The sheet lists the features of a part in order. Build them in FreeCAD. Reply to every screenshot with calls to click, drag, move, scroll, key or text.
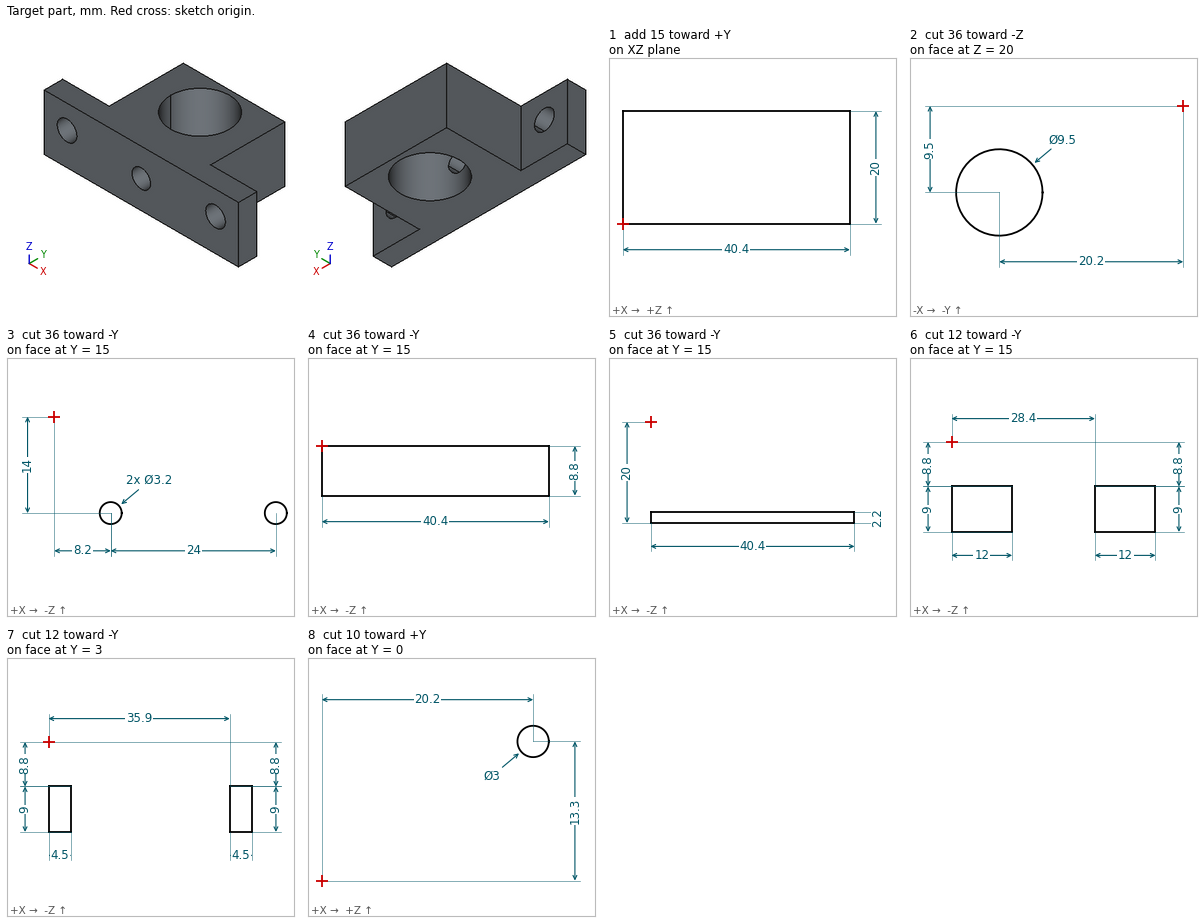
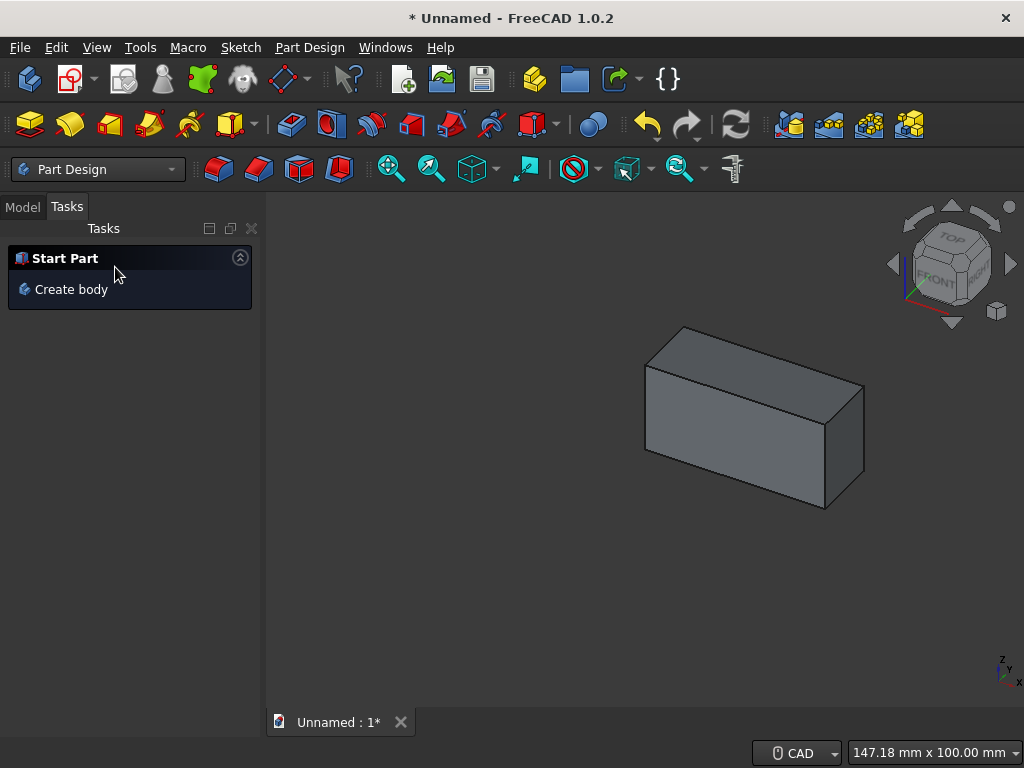
key(v)
key(f)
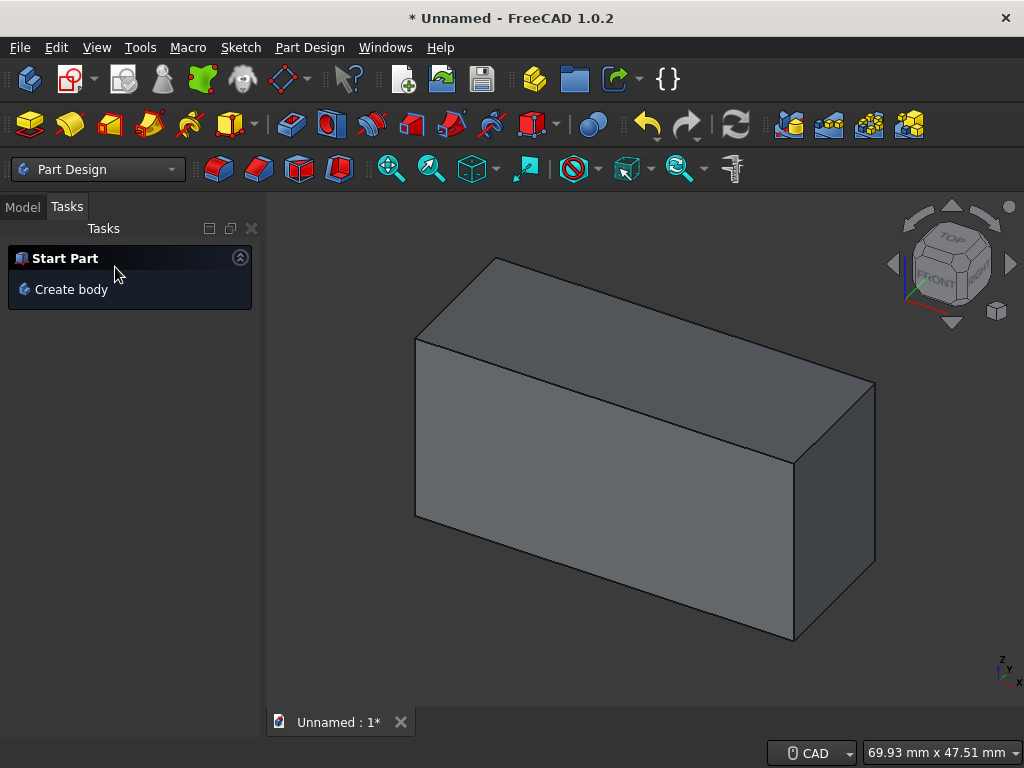
click(753, 396)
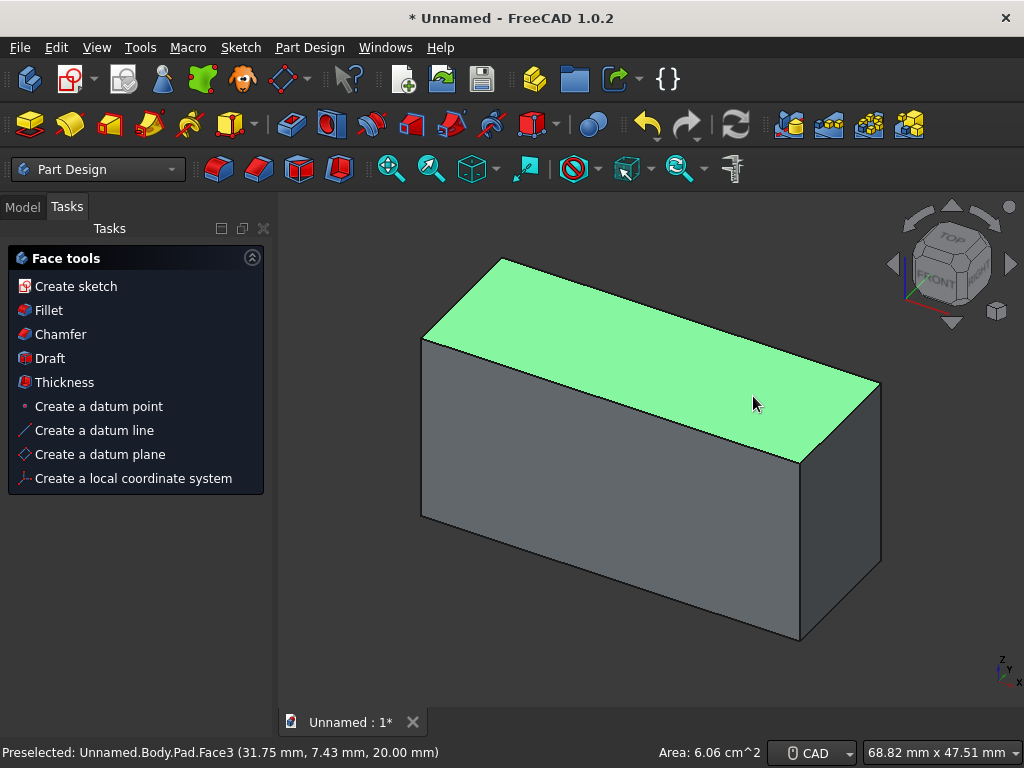
click(70, 80)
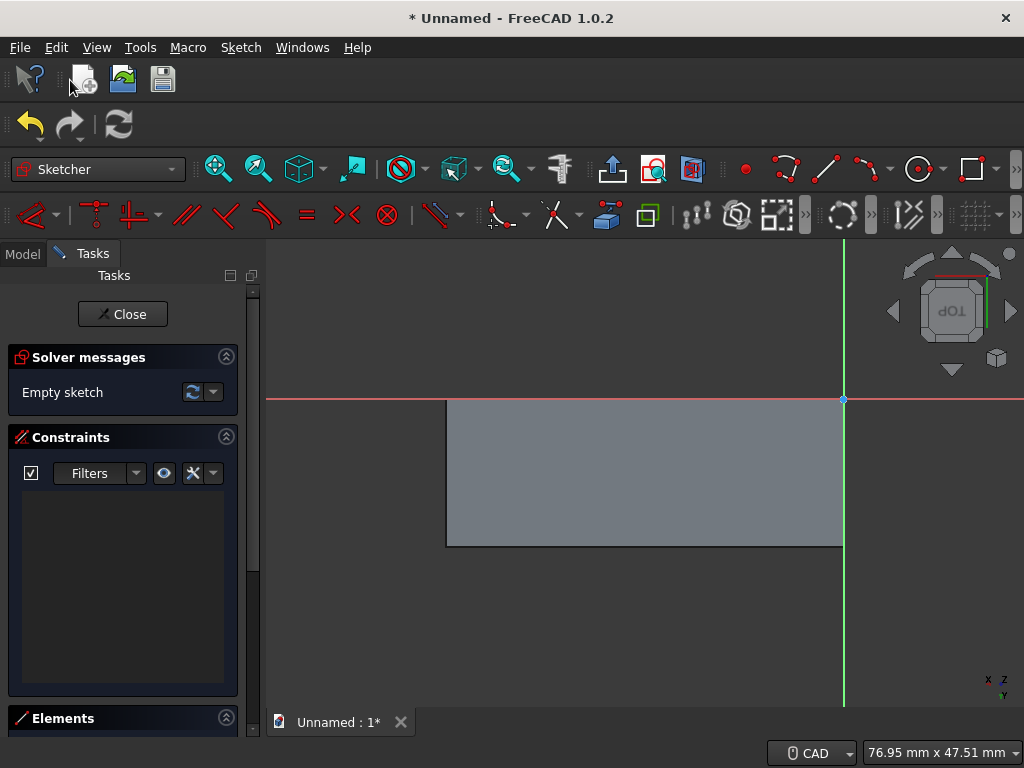
scroll(675, 501, up, 6)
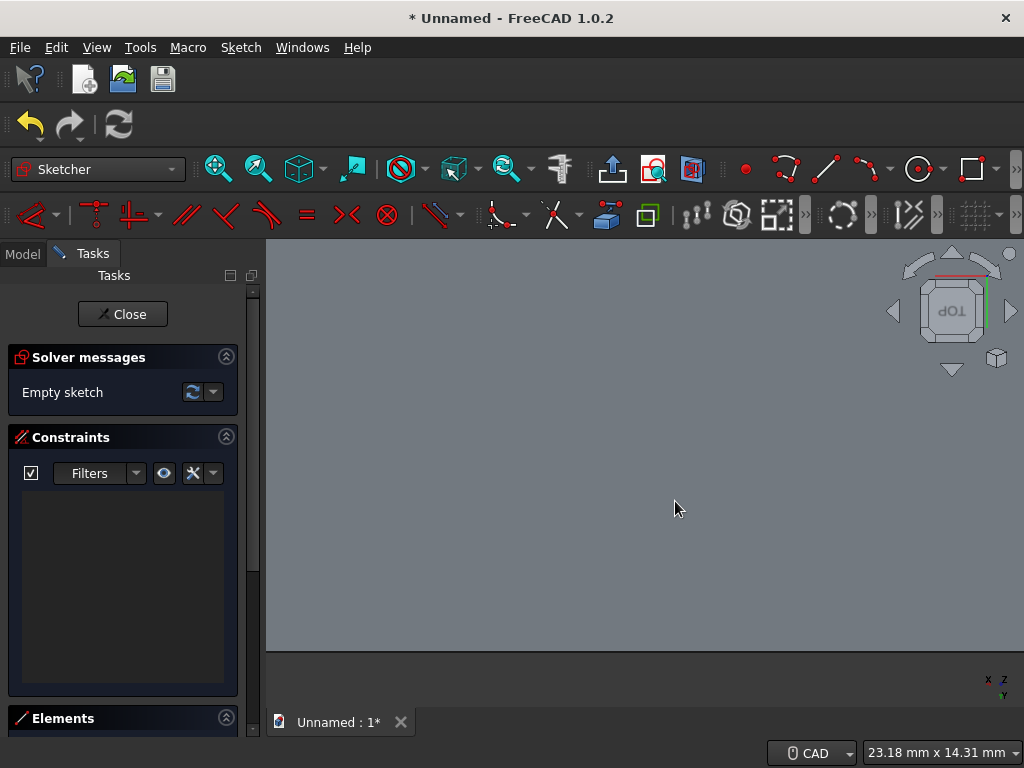
click(920, 170)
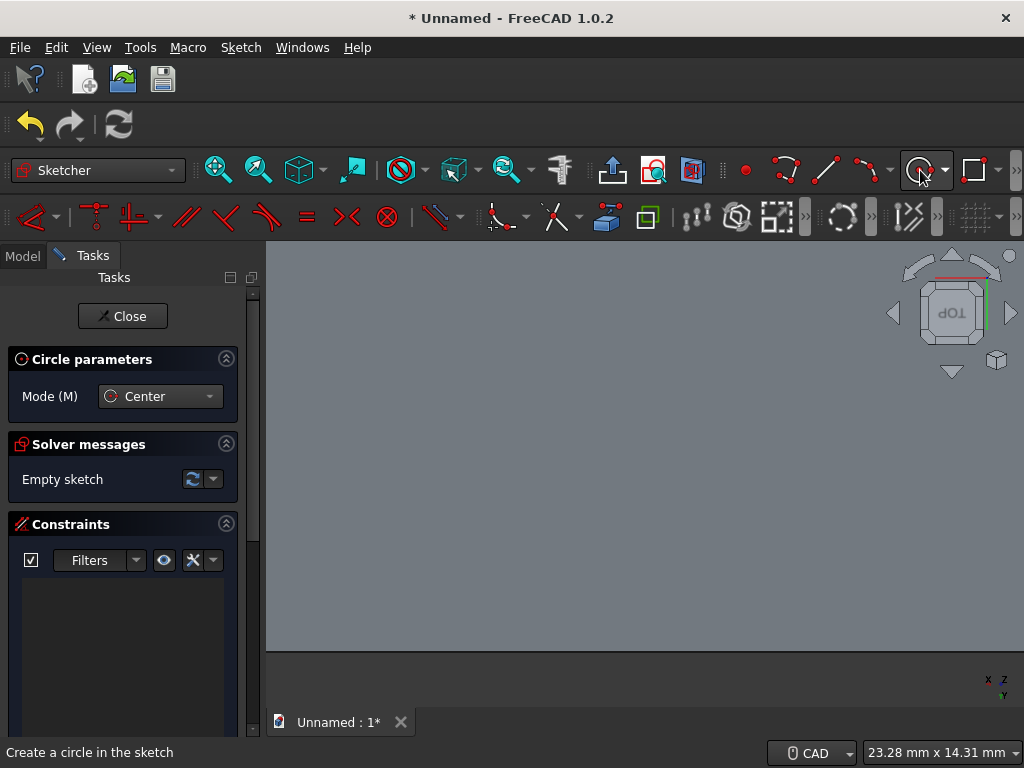
click(574, 473)
move(684, 364)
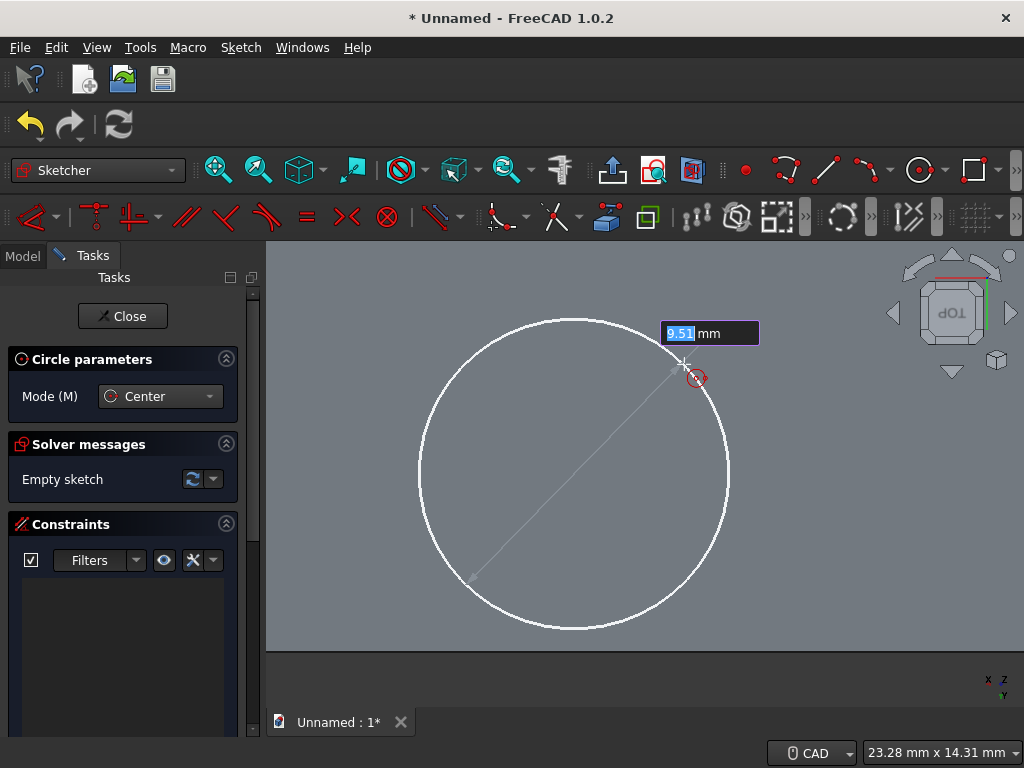
text(9.5)
key(Return)
key(Escape)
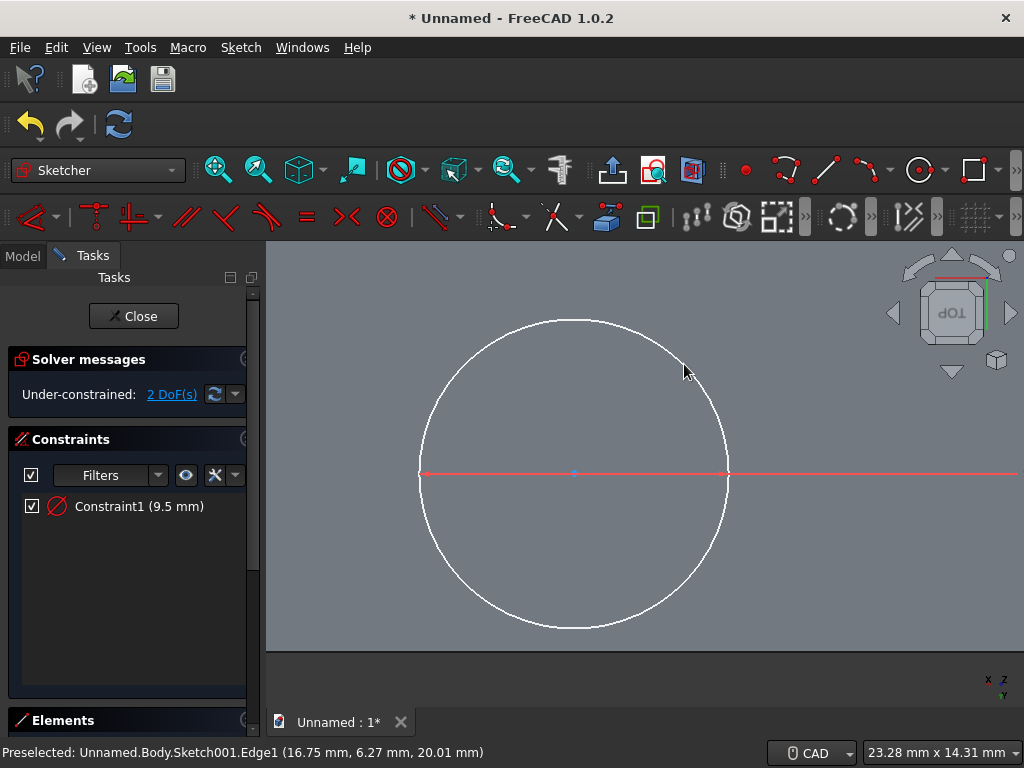
click(574, 474)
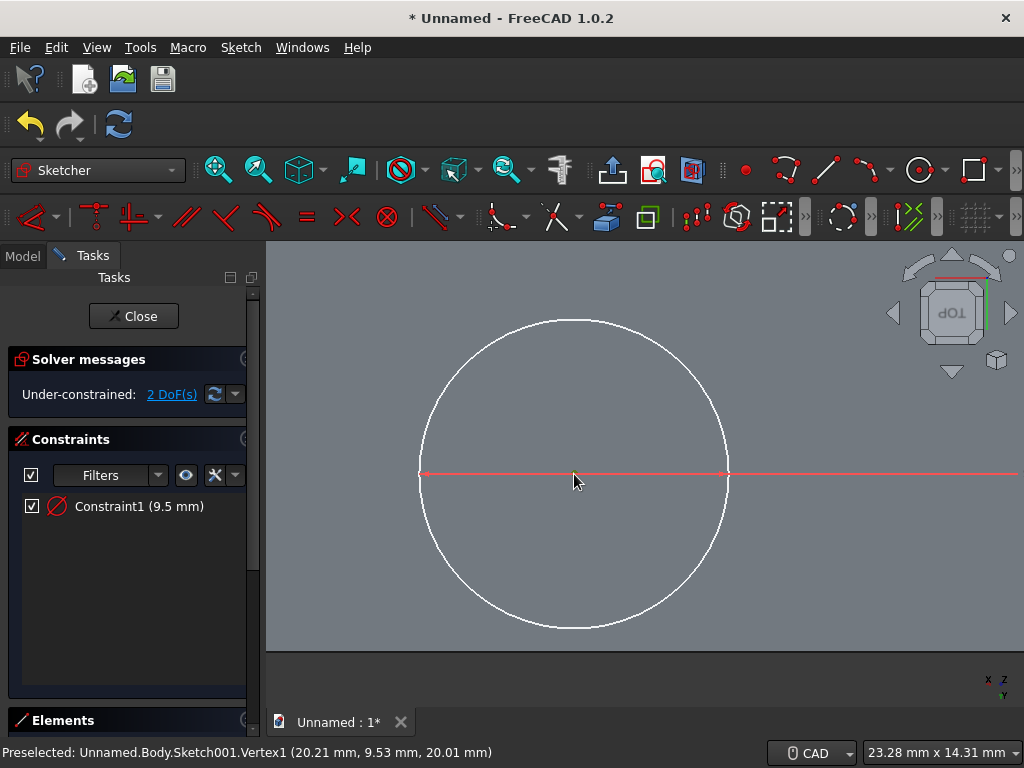
key(i)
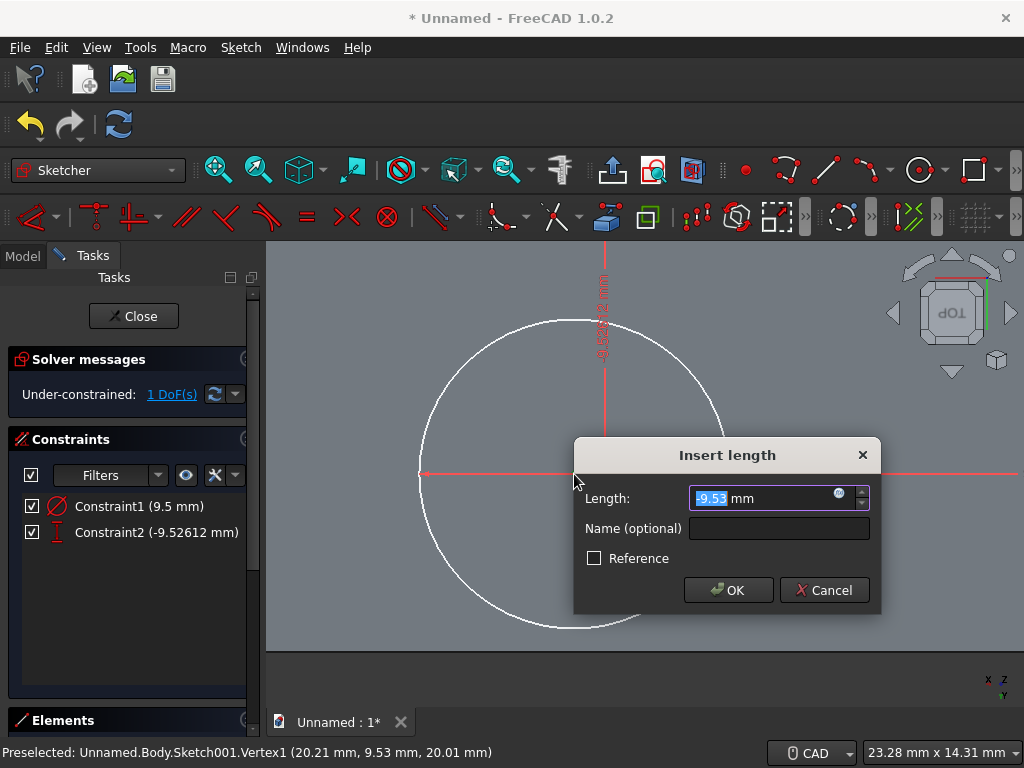
text(-9.5)
key(Return)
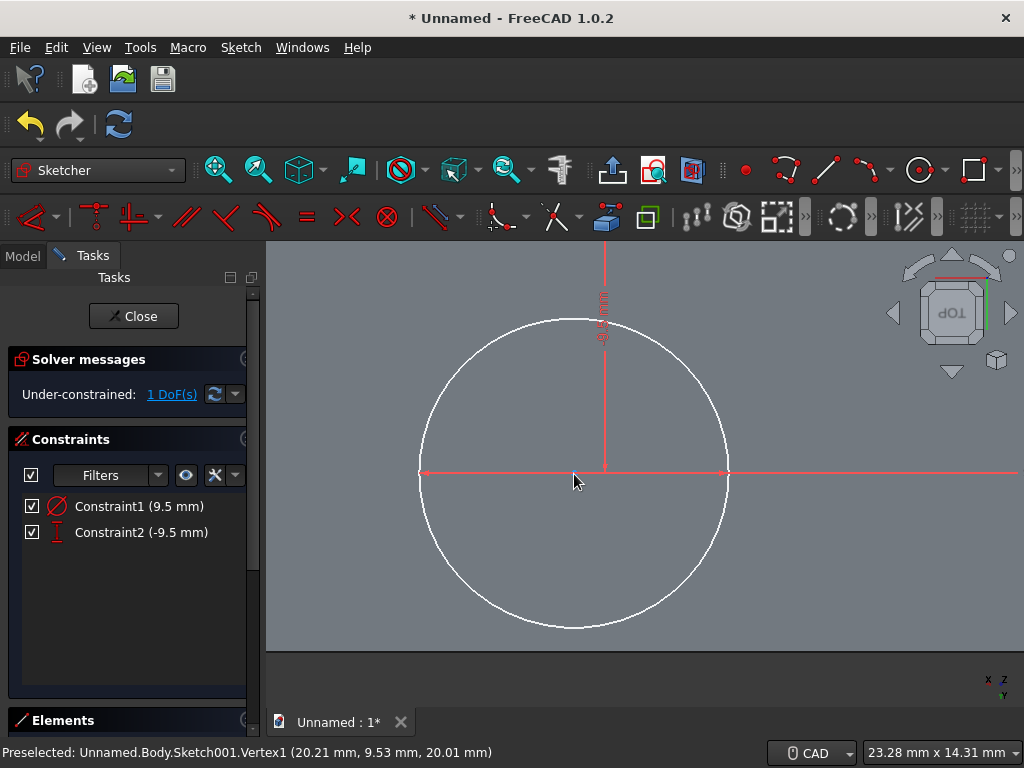
click(574, 473)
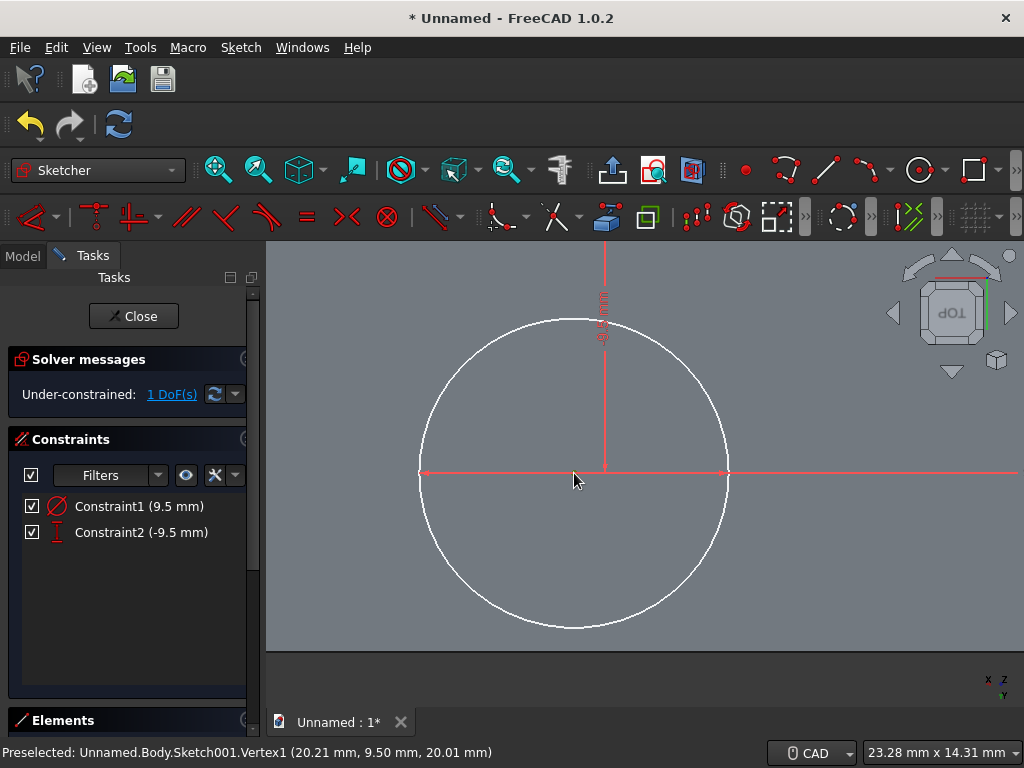
key(l)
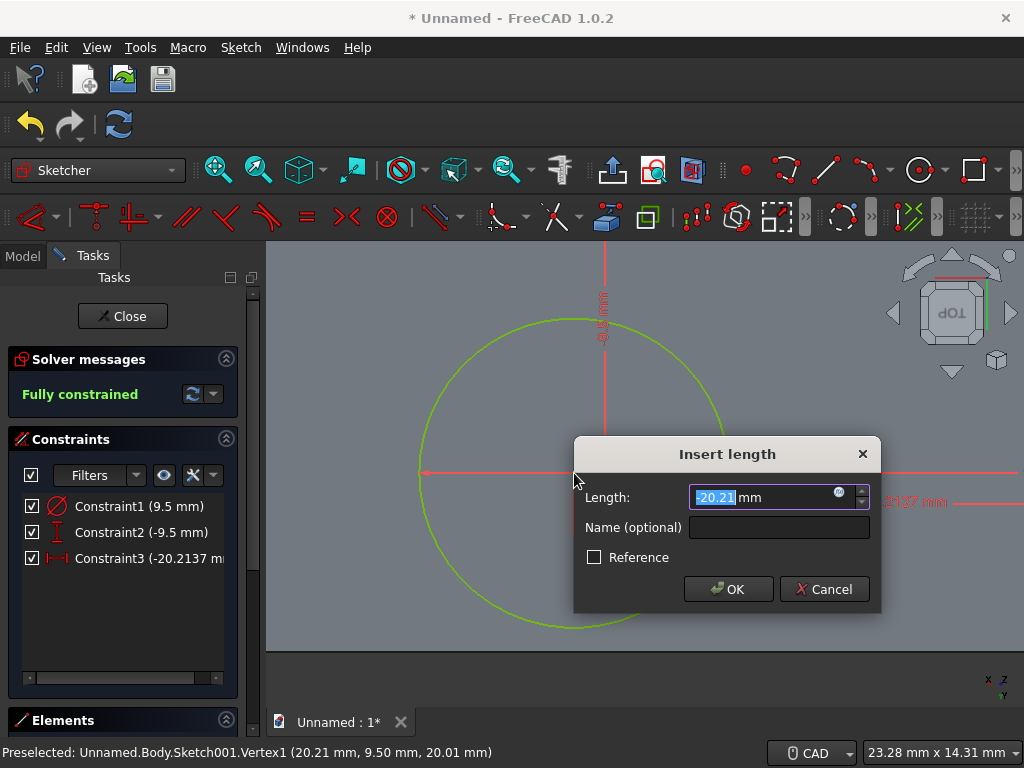
text(-20.2)
key(Return)